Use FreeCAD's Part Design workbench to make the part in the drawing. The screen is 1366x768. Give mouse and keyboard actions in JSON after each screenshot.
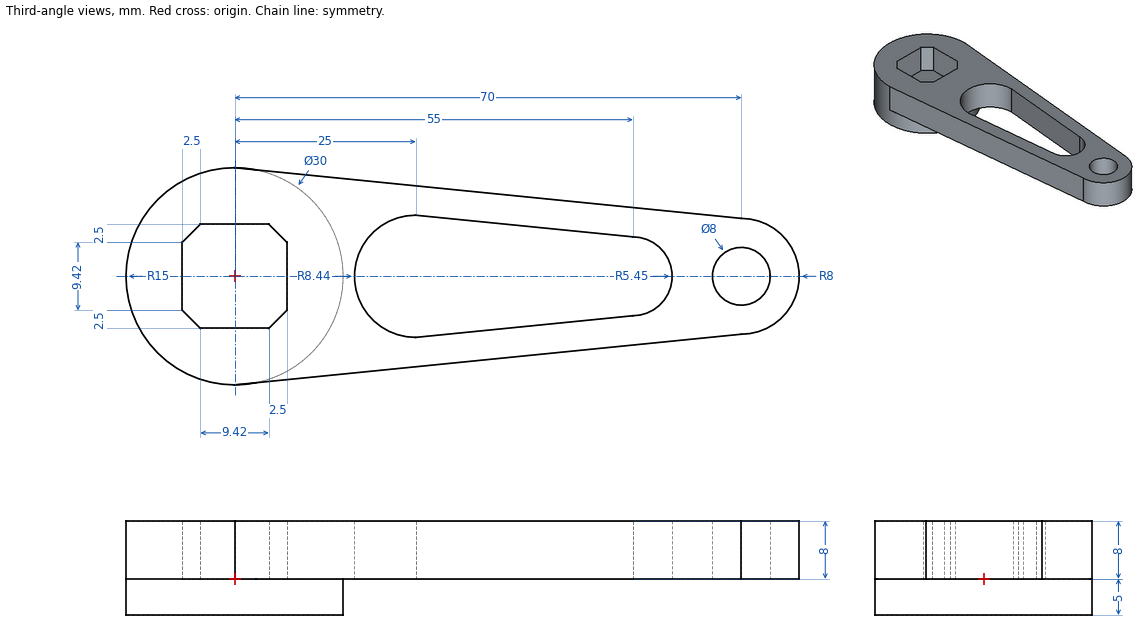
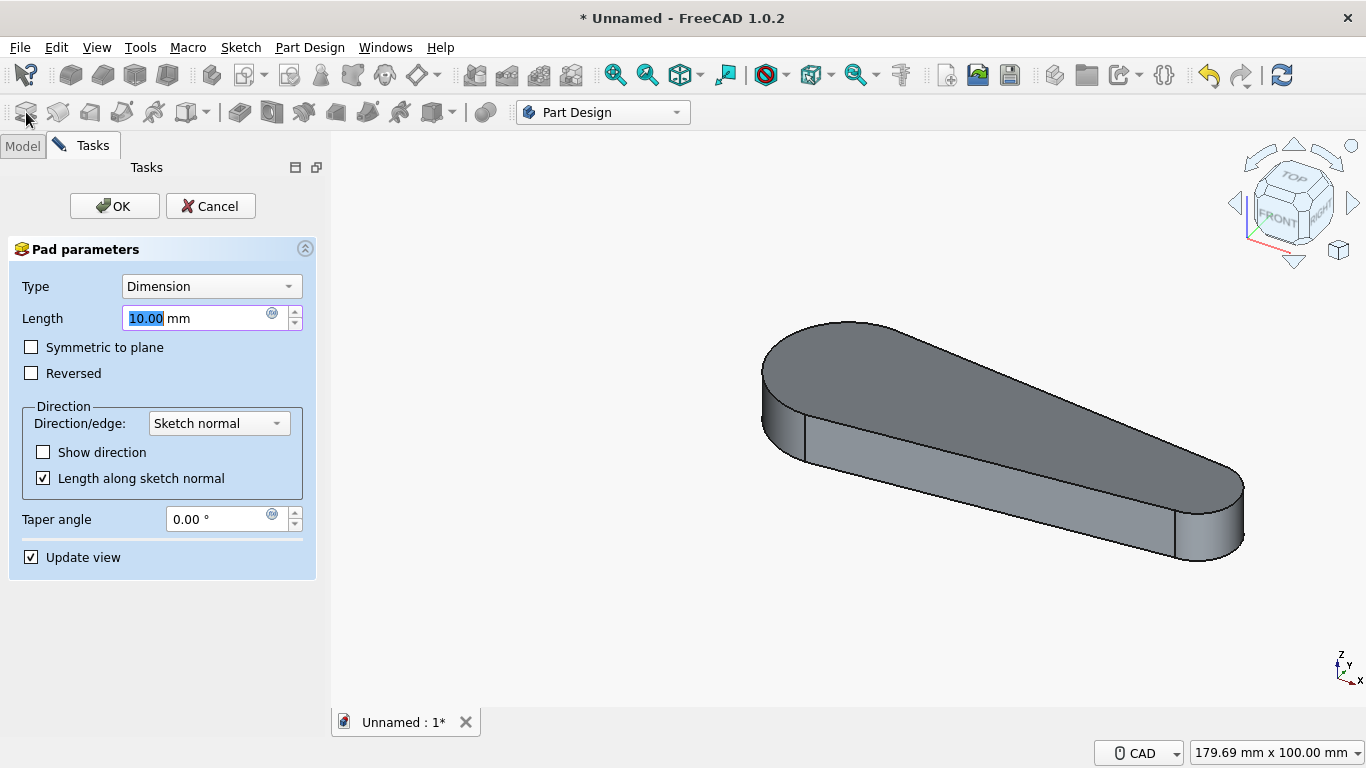
{"action": "type", "text": "8"}
{"action": "key", "text": "Tab"}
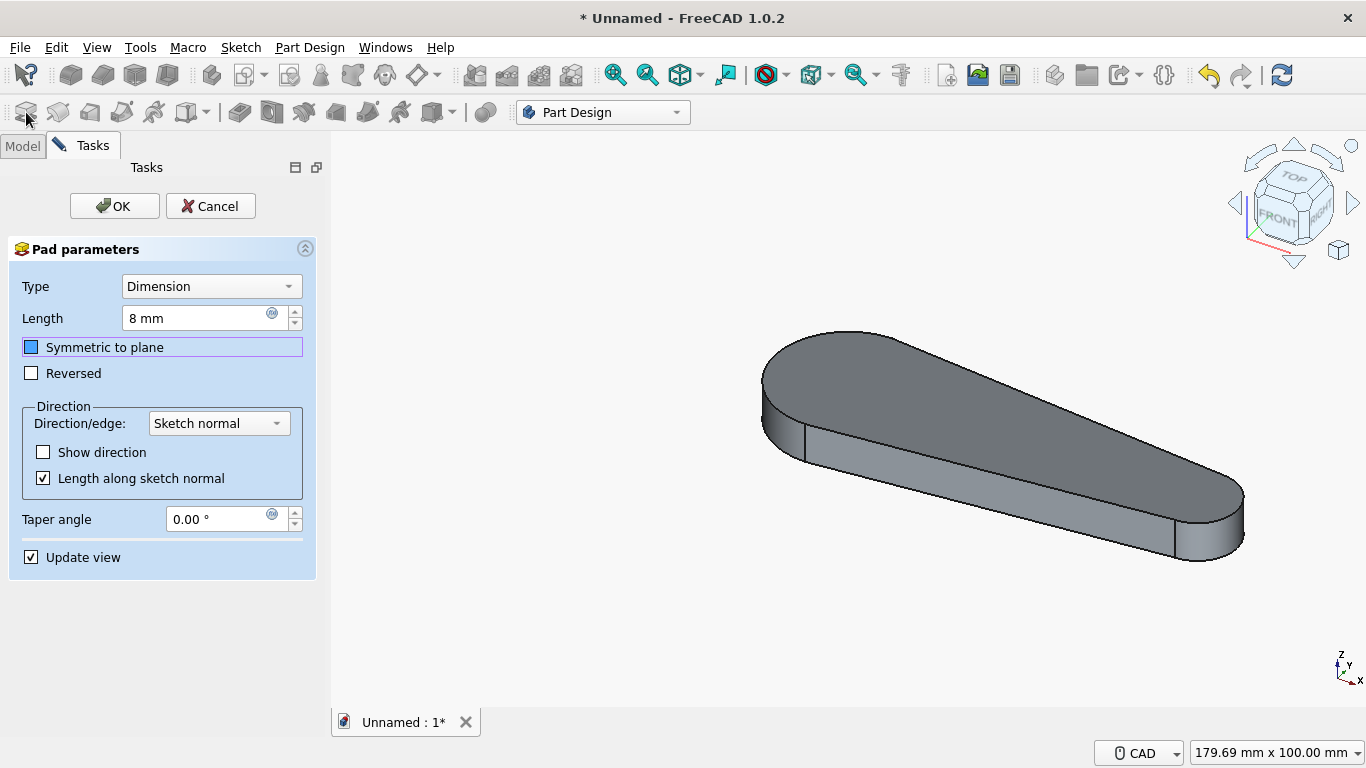
{"action": "left_click", "coordinate": [115, 206]}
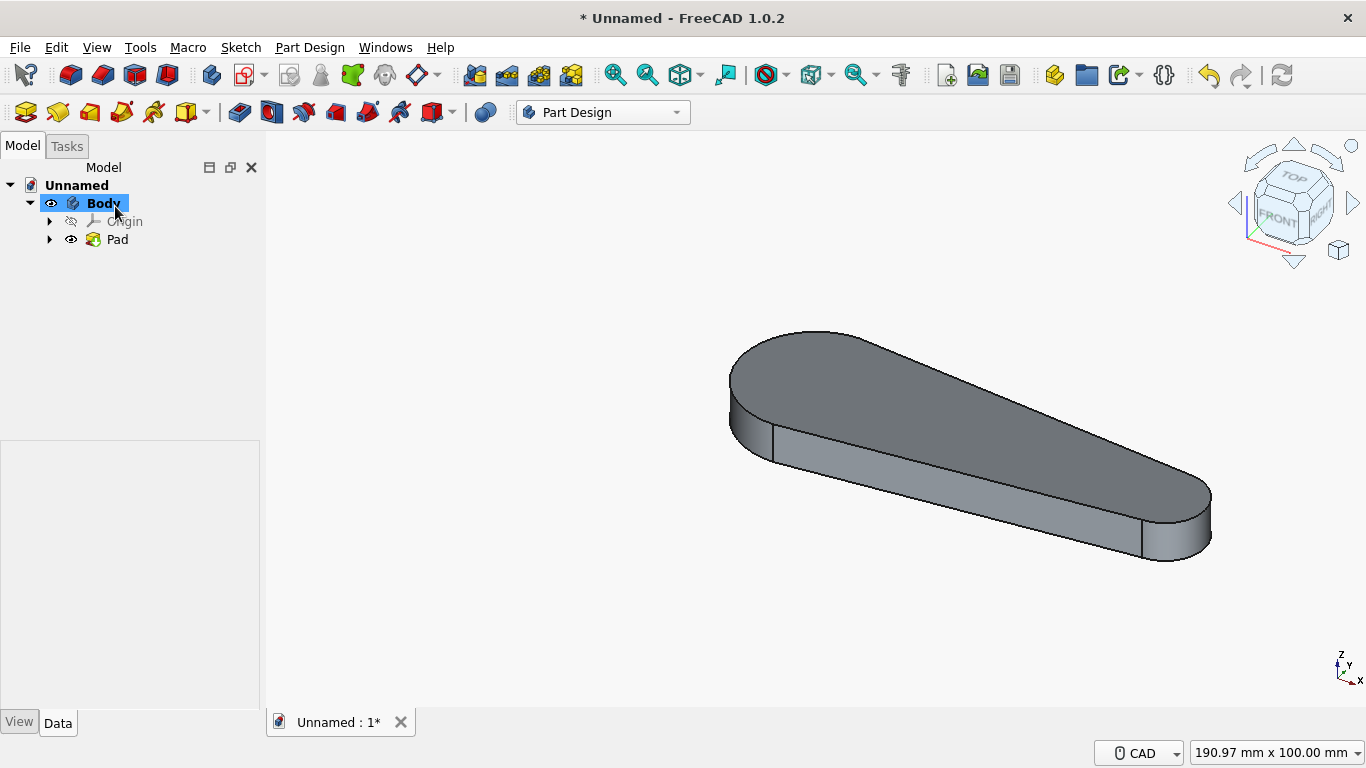
{"action": "left_click", "coordinate": [841, 388]}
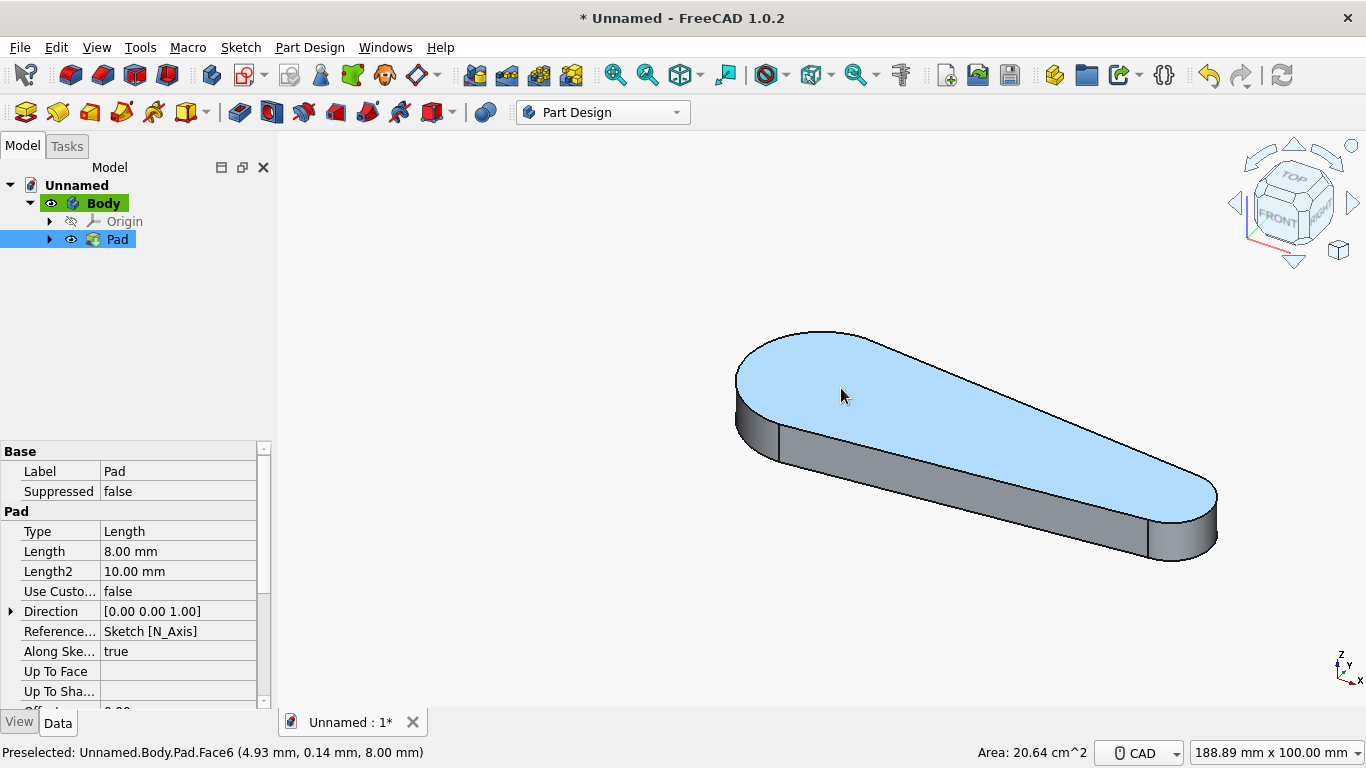
{"action": "left_click", "coordinate": [244, 76]}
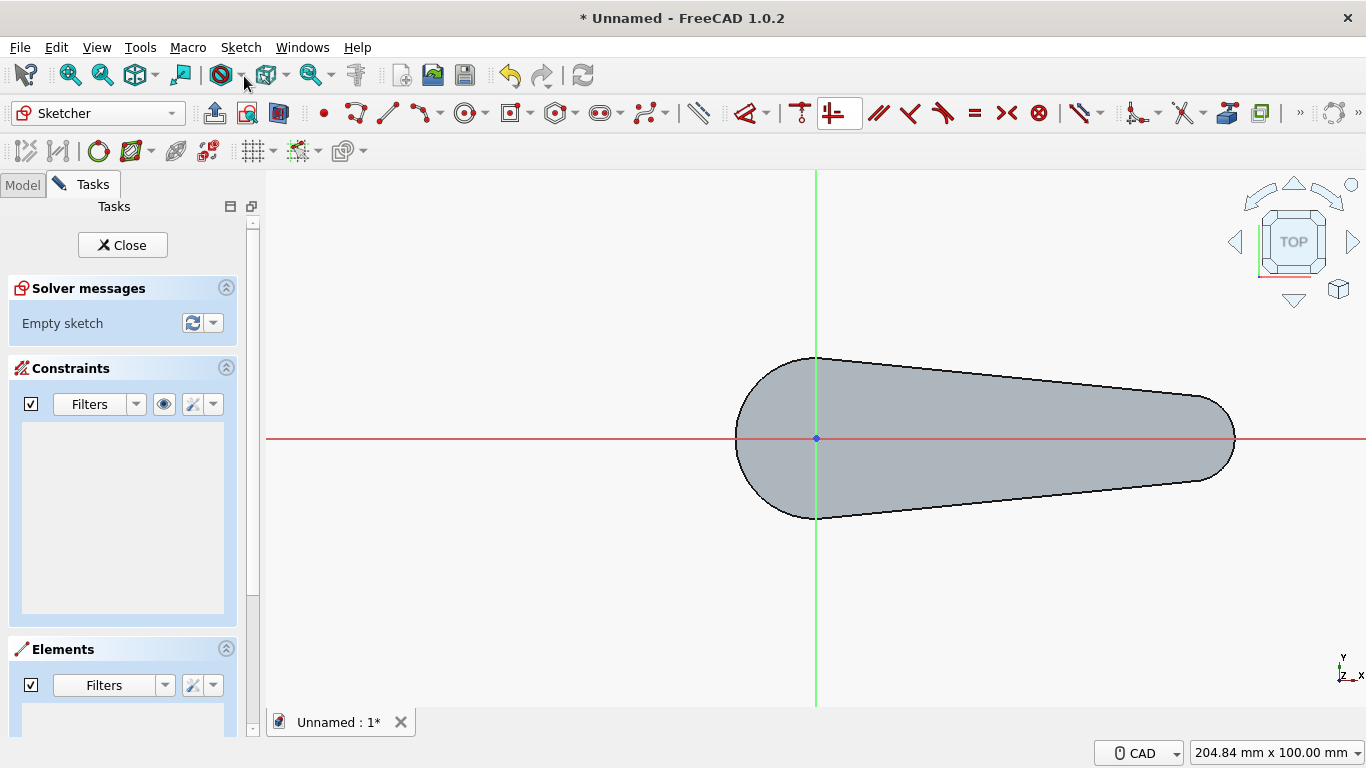
{"action": "scroll", "coordinate": [1201, 438], "scroll_direction": "up", "scroll_amount": 3}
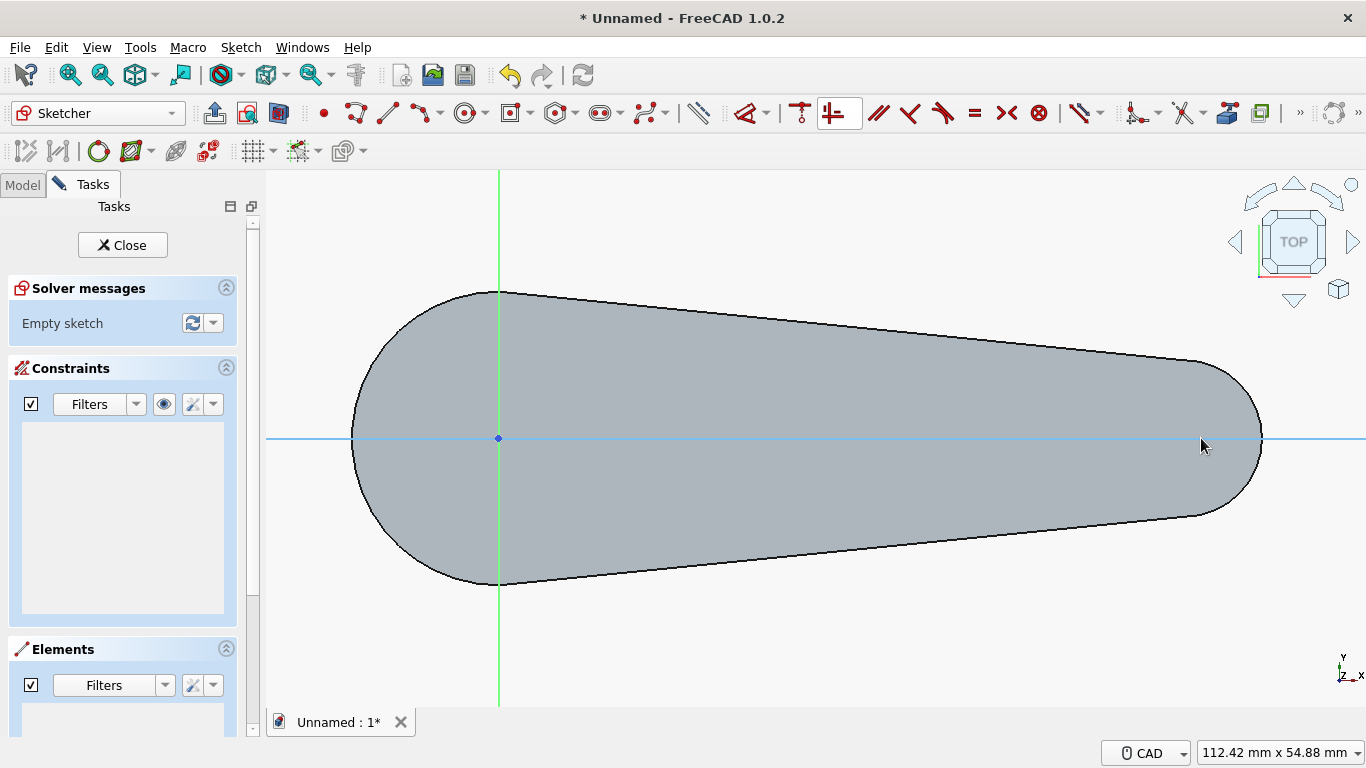
{"action": "left_click", "coordinate": [388, 114]}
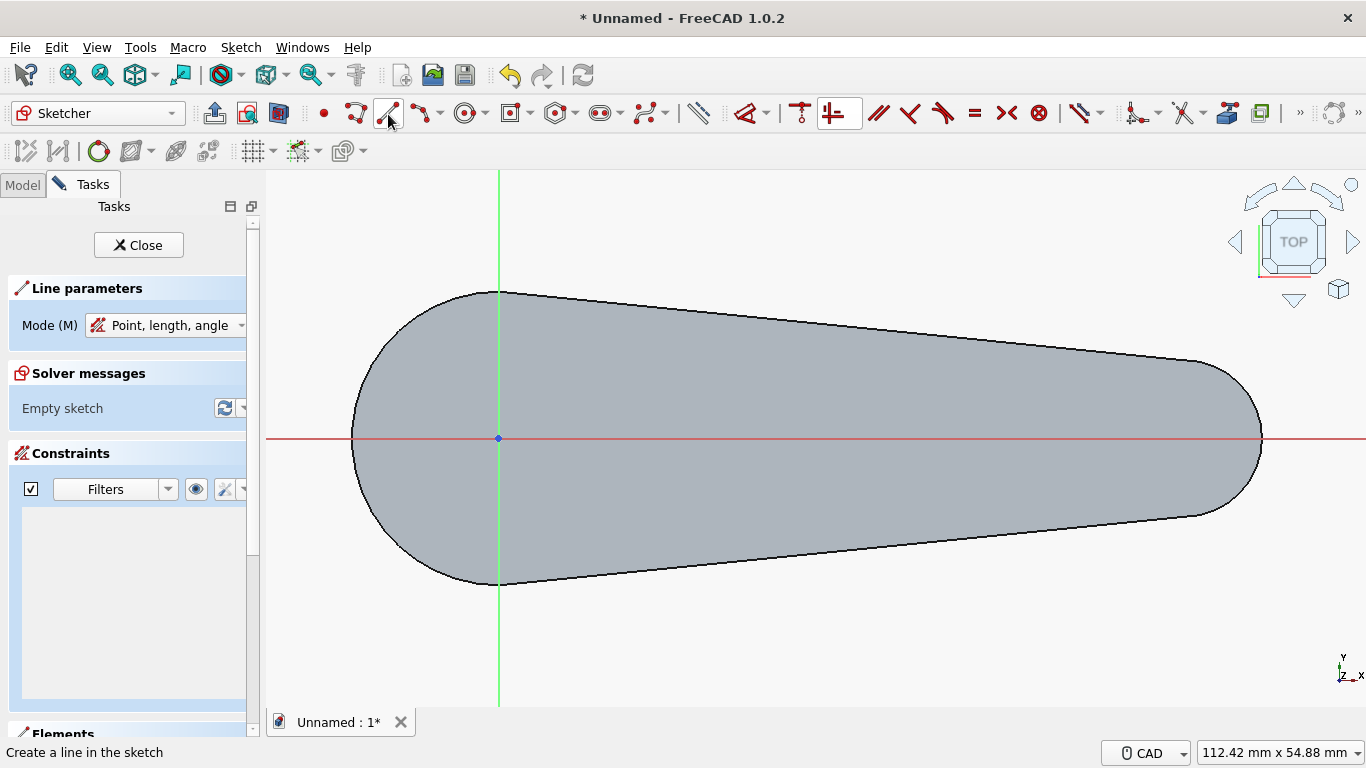
{"action": "left_click", "coordinate": [1037, 385]}
{"action": "left_click", "coordinate": [743, 356]}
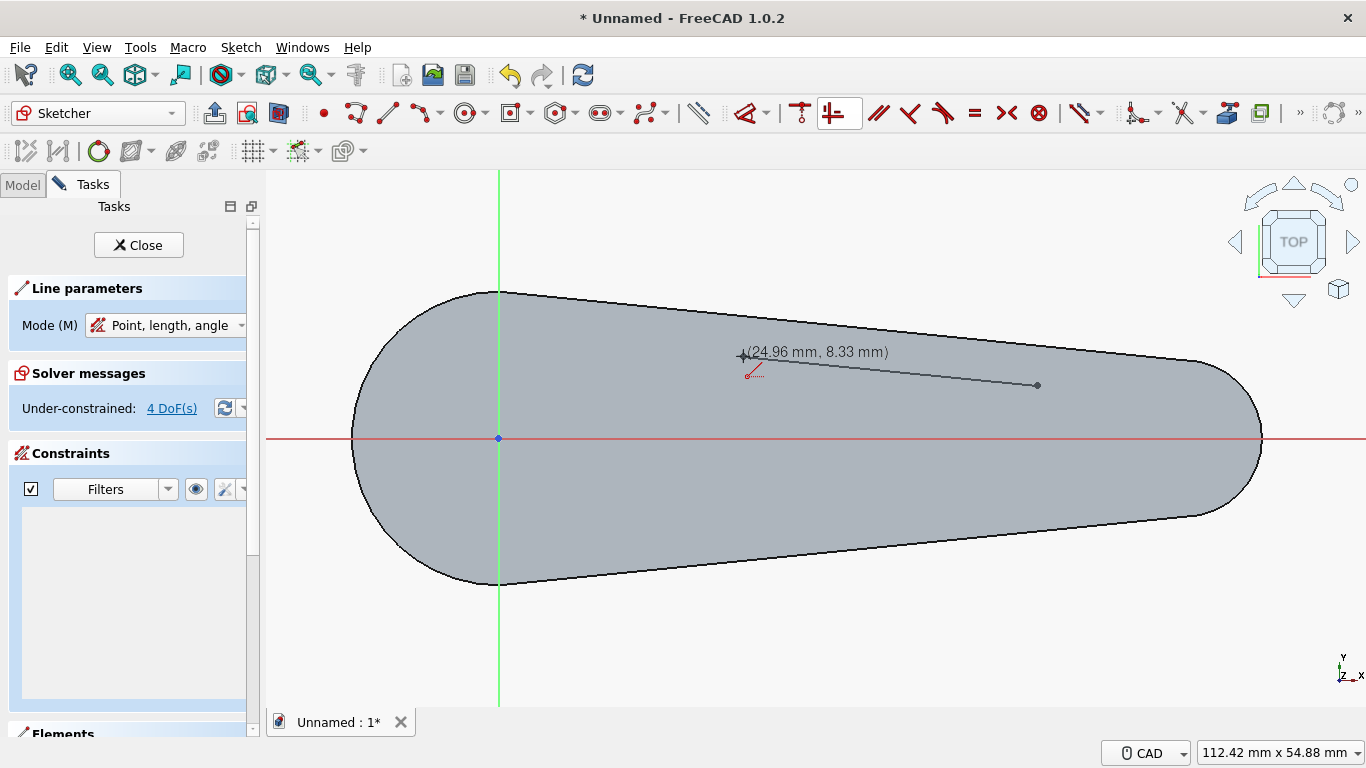
{"action": "left_click", "coordinate": [743, 521]}
{"action": "left_click", "coordinate": [1037, 492]}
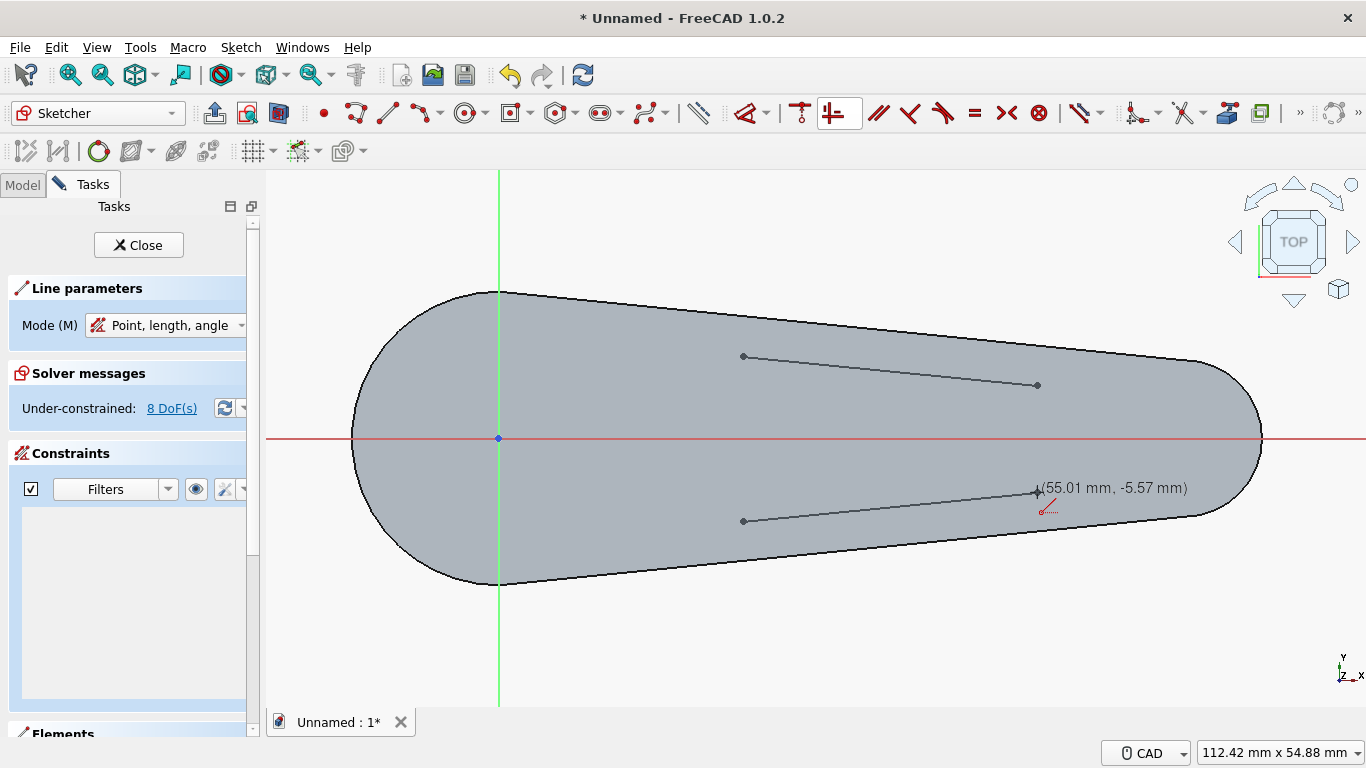
{"action": "key", "text": "g 3 a"}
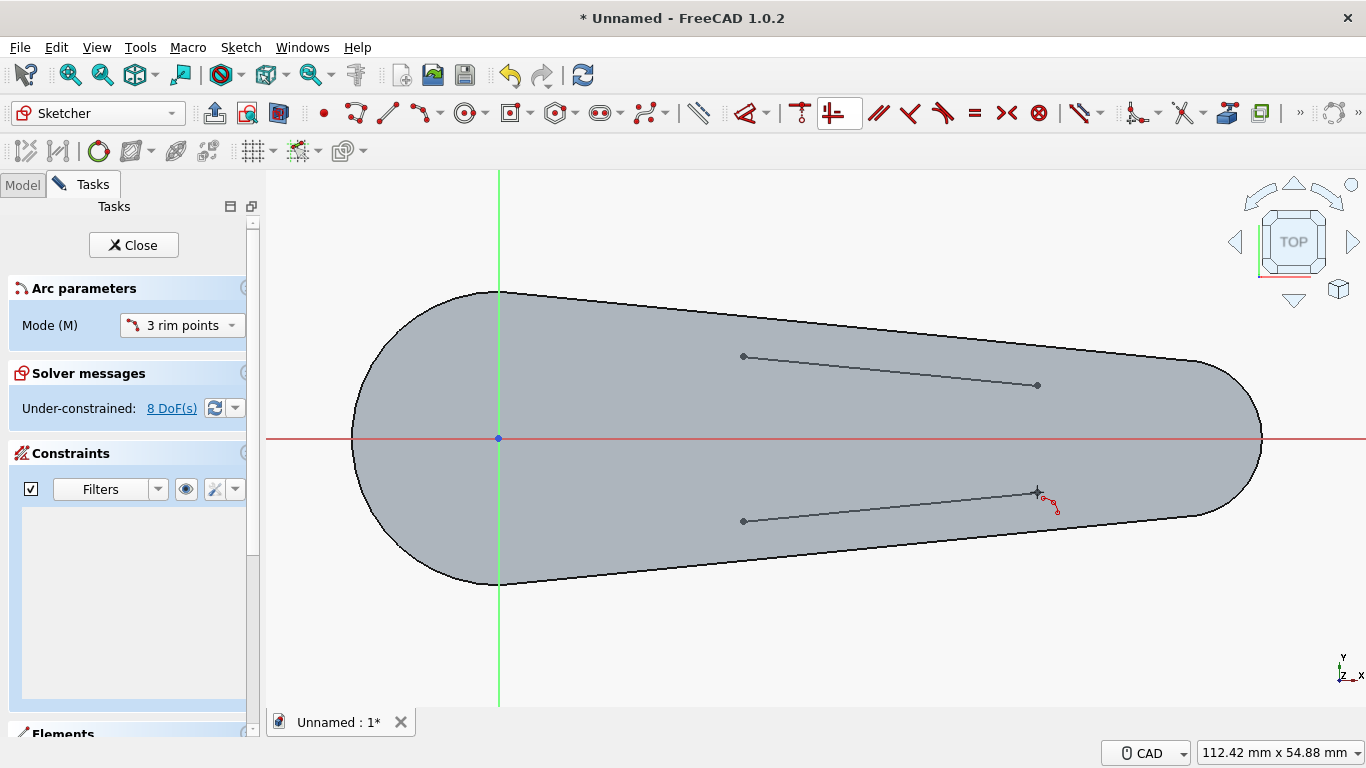
{"action": "left_click", "coordinate": [743, 357]}
{"action": "left_click", "coordinate": [743, 522]}
{"action": "left_click", "coordinate": [665, 413]}